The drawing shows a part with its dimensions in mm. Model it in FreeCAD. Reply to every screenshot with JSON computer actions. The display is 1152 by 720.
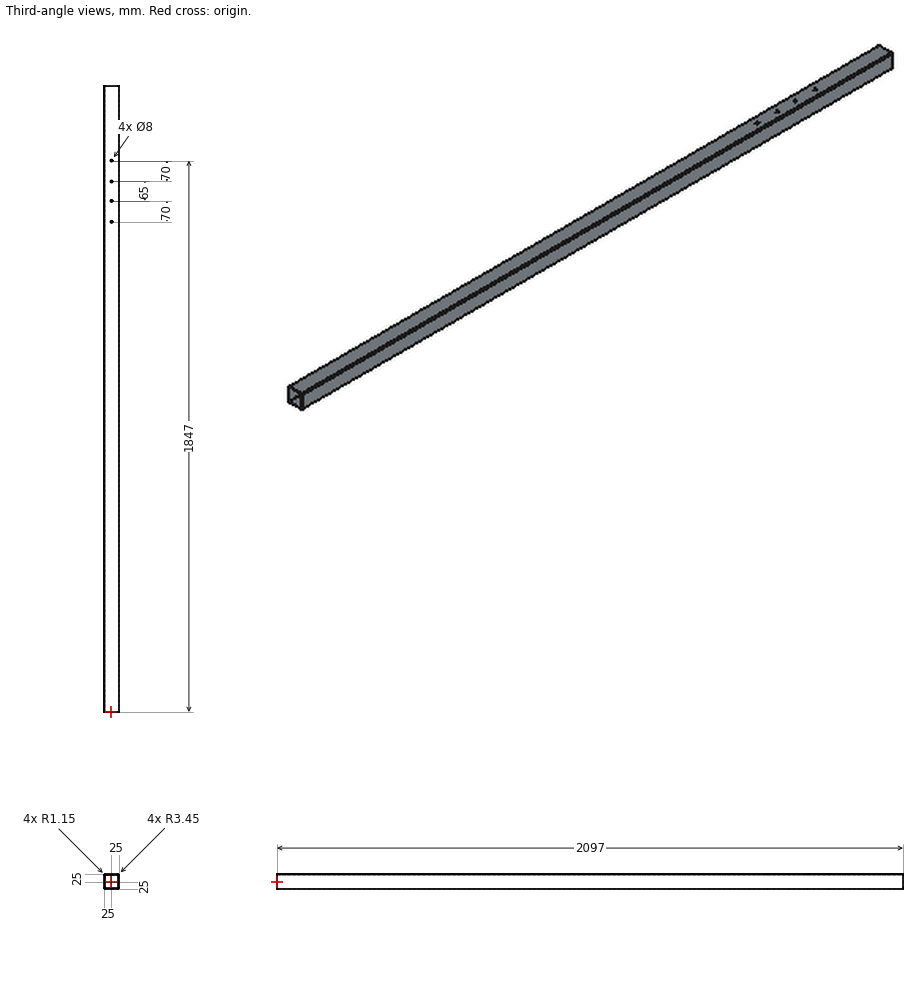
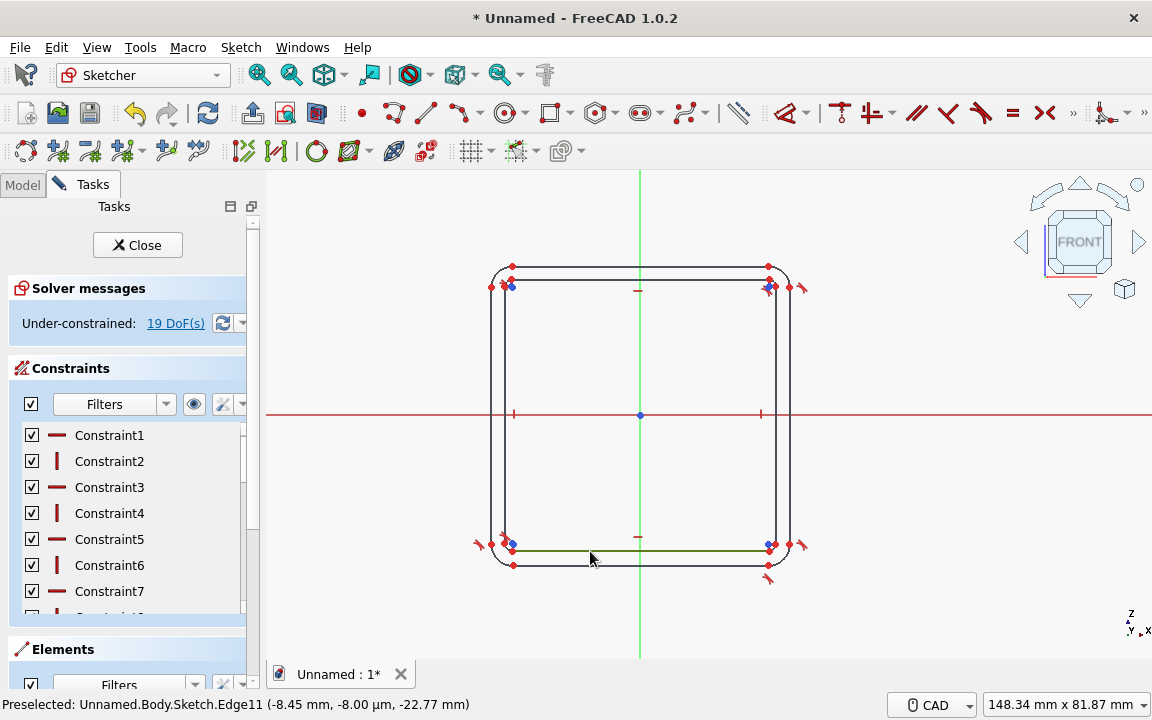
{"action": "scroll", "coordinate": [774, 549], "scroll_direction": "up", "scroll_amount": 5}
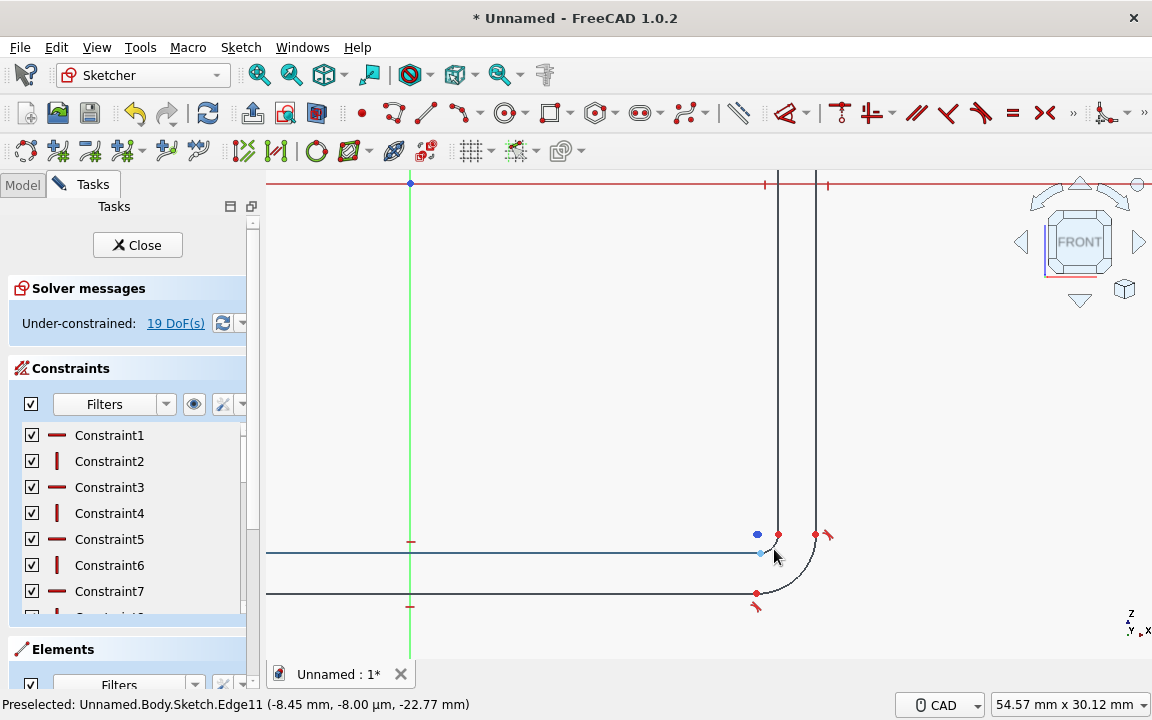
{"action": "left_click", "coordinate": [773, 547]}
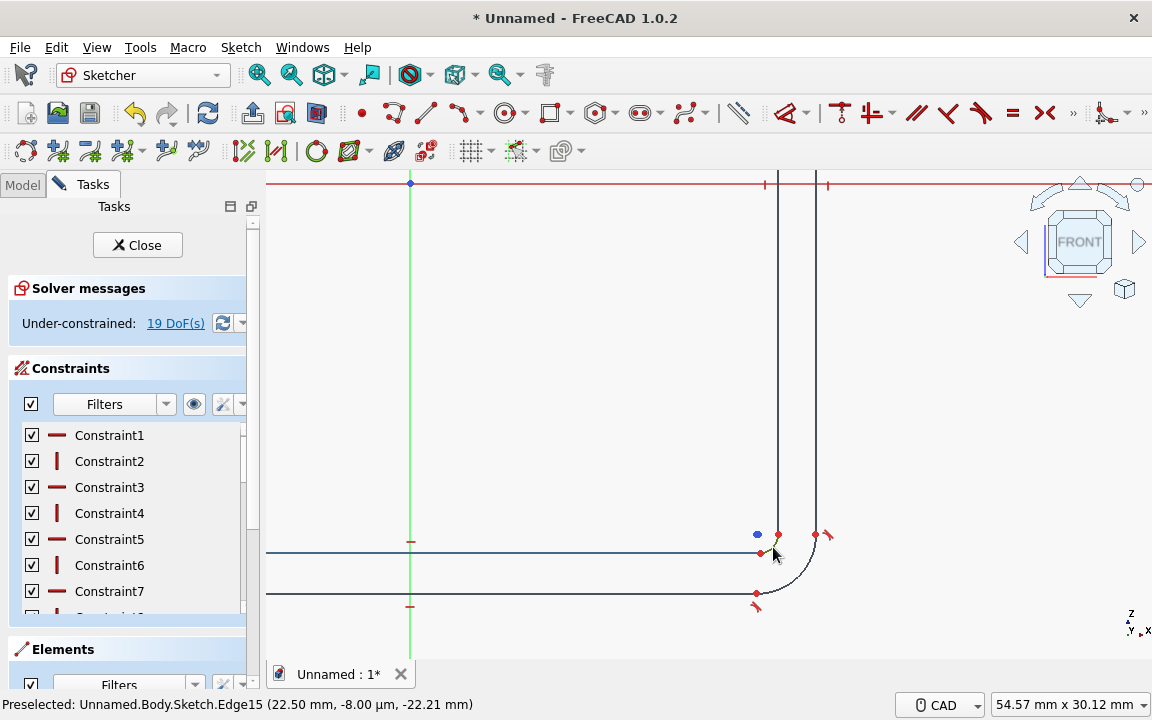
{"action": "left_click", "coordinate": [982, 114]}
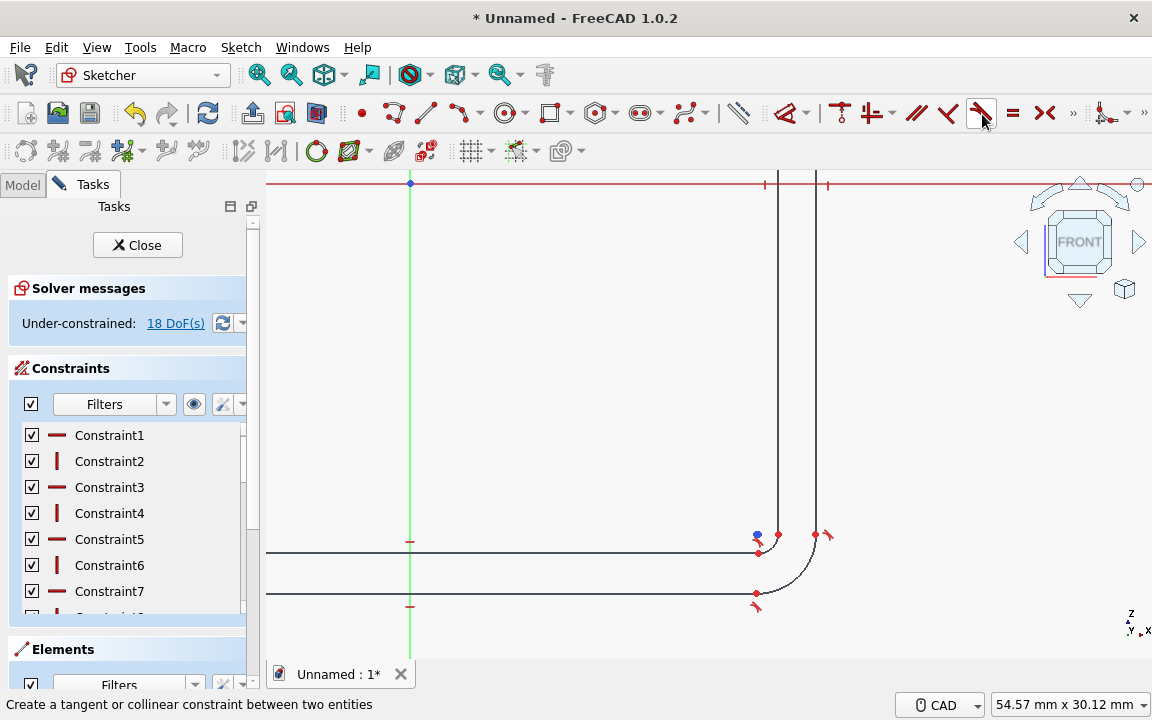
{"action": "left_click", "coordinate": [778, 325]}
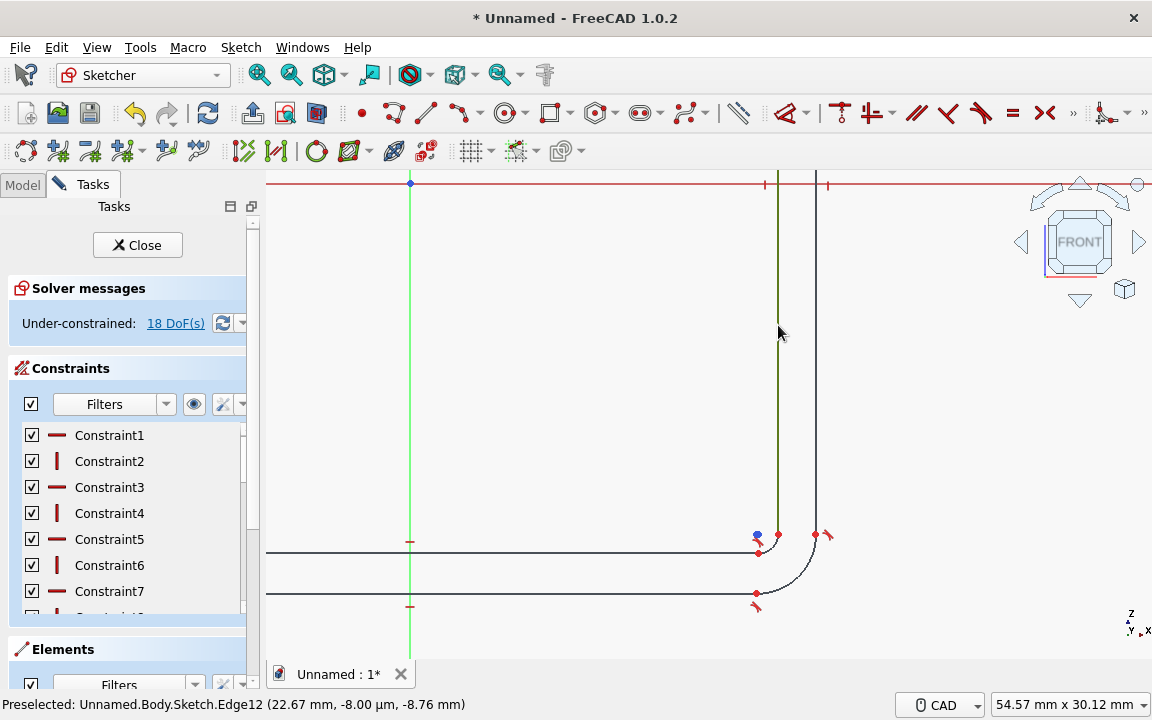
{"action": "left_click", "coordinate": [772, 548]}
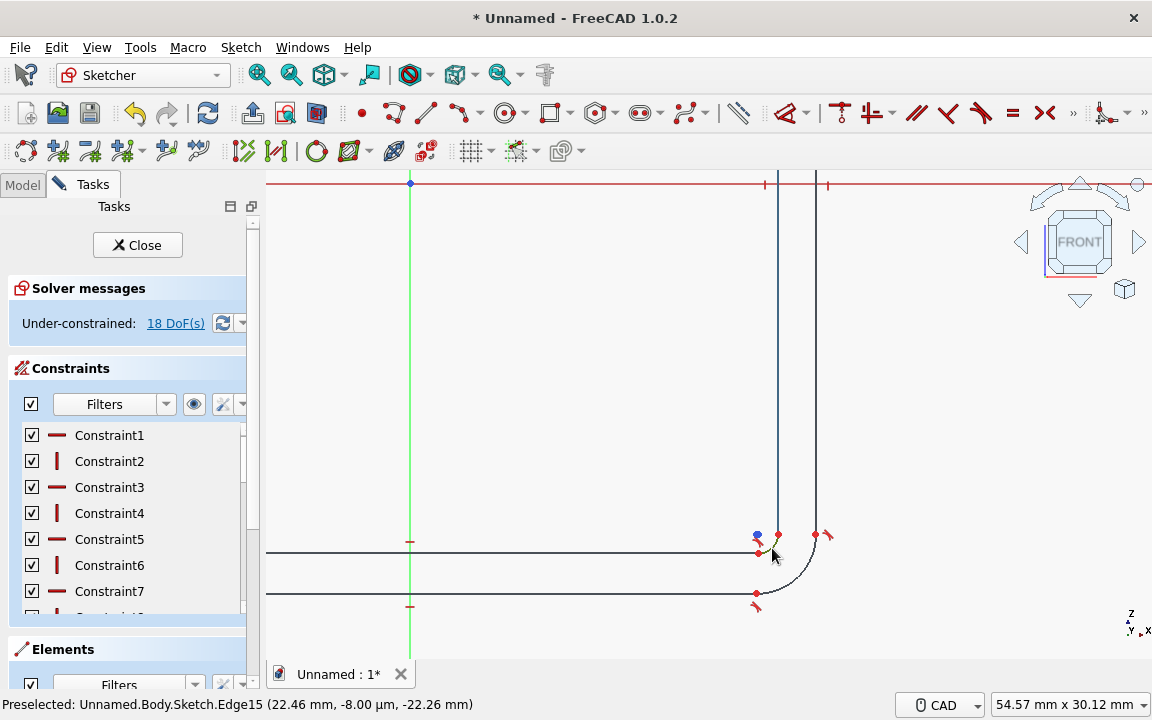
{"action": "left_click", "coordinate": [982, 114]}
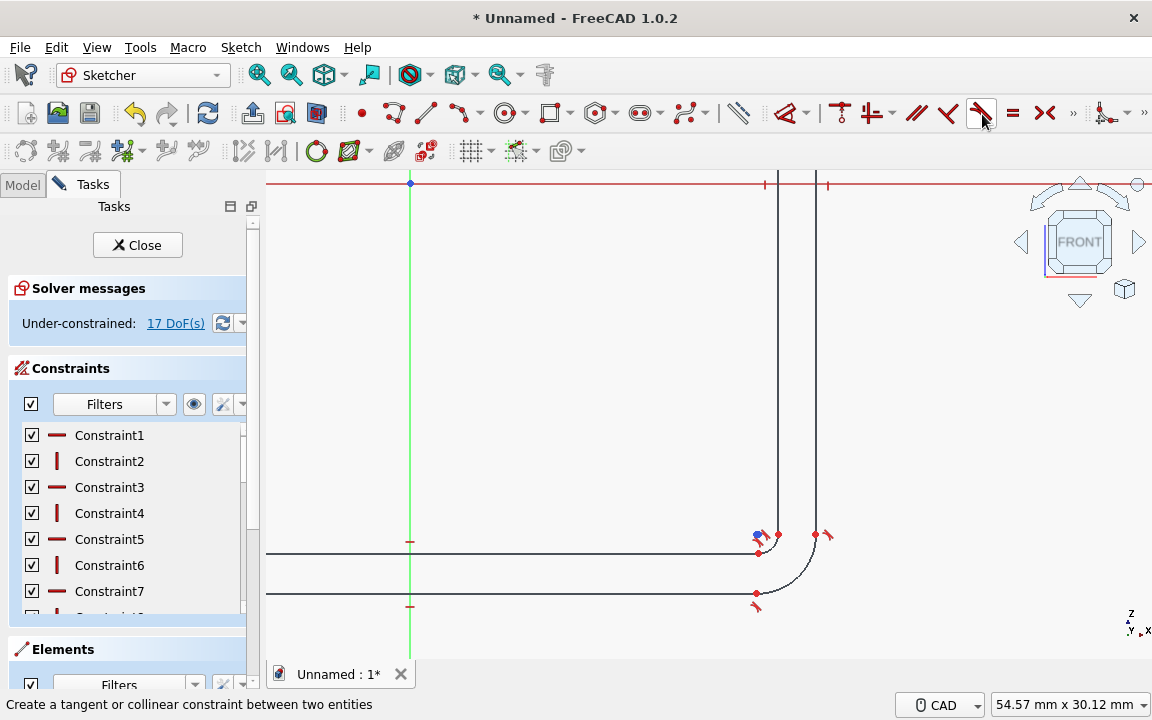
{"action": "left_click", "coordinate": [778, 325]}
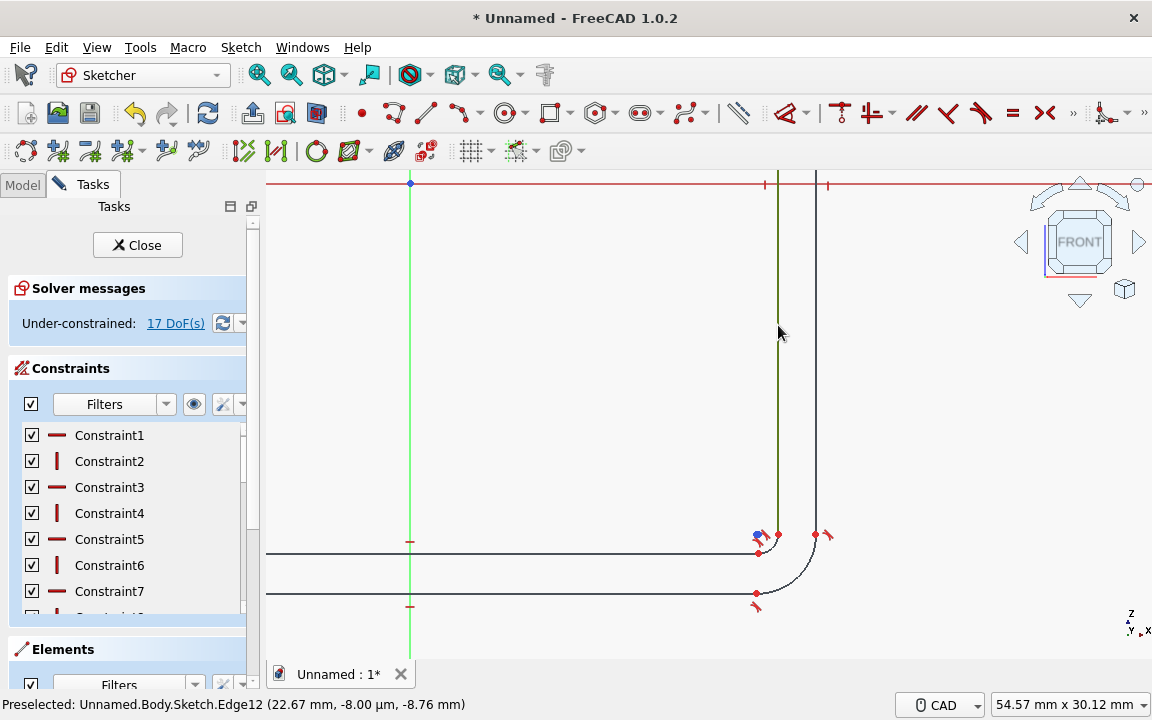
{"action": "scroll", "coordinate": [775, 549], "scroll_direction": "down", "scroll_amount": 5}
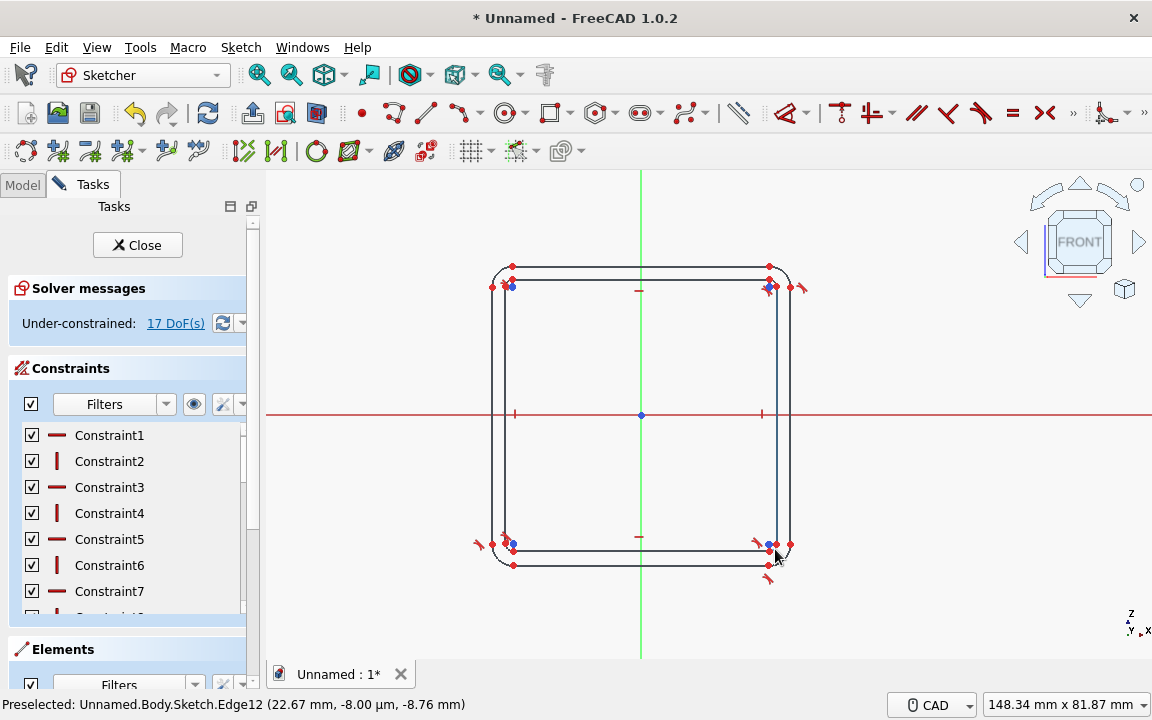
{"action": "scroll", "coordinate": [775, 282], "scroll_direction": "up", "scroll_amount": 5}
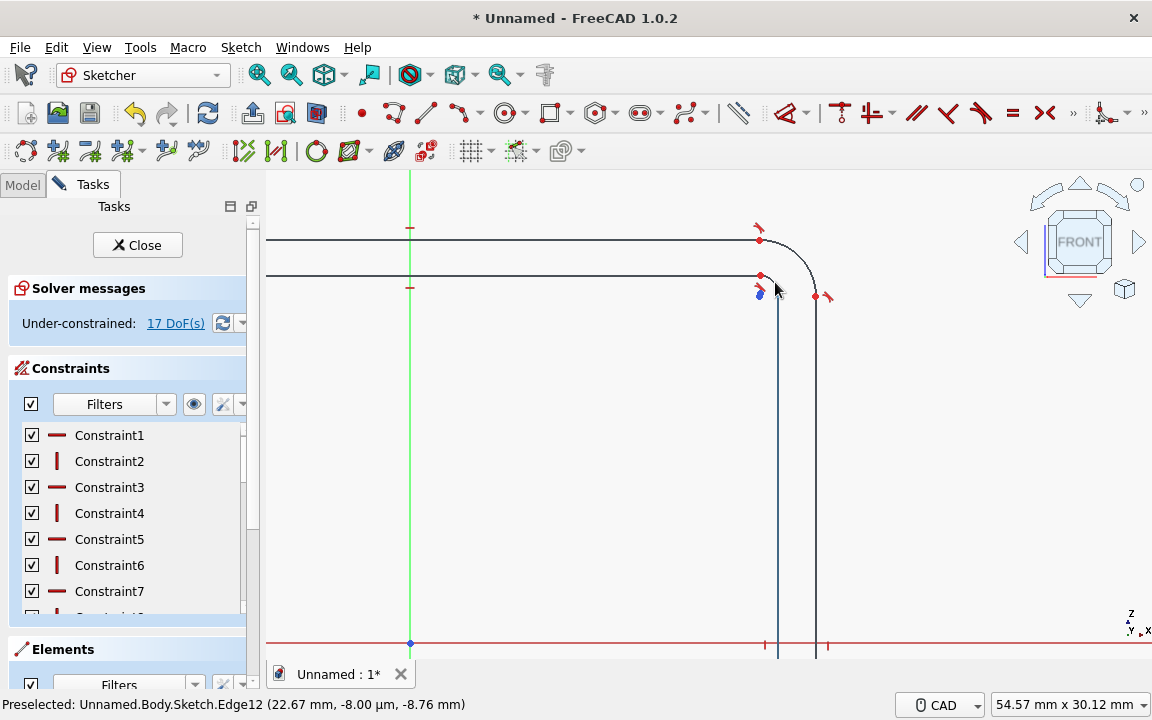
{"action": "left_click", "coordinate": [773, 281]}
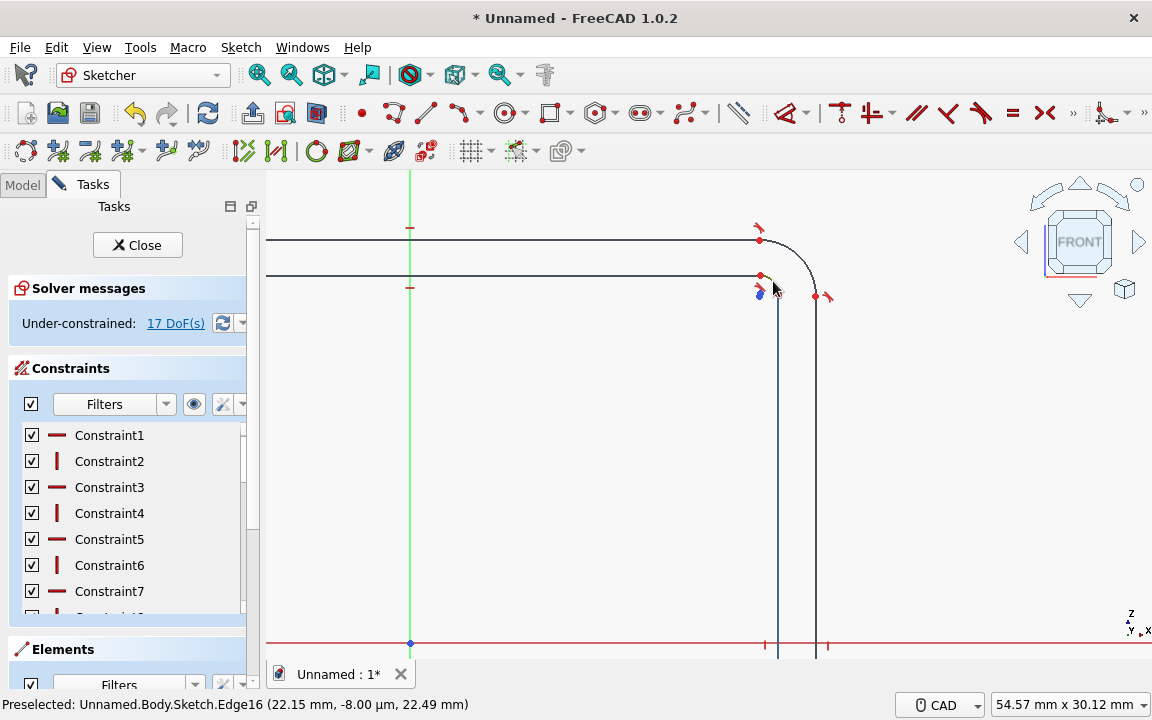
{"action": "left_click", "coordinate": [982, 114]}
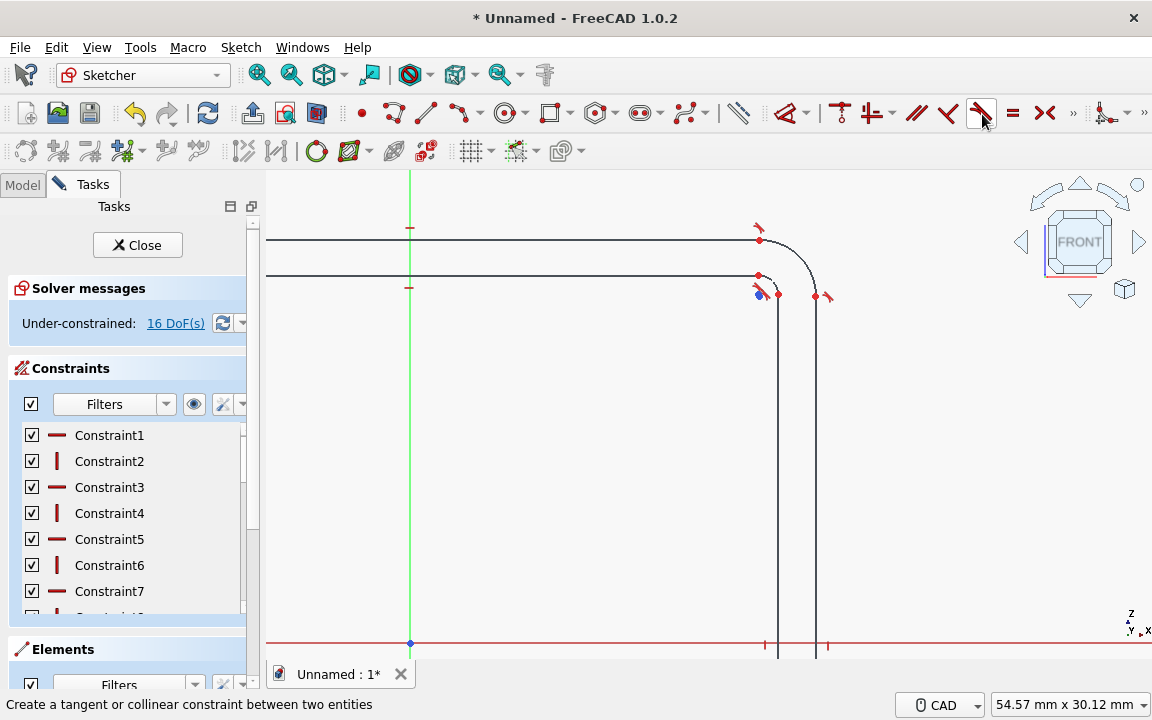
{"action": "scroll", "coordinate": [775, 281], "scroll_direction": "down", "scroll_amount": 5}